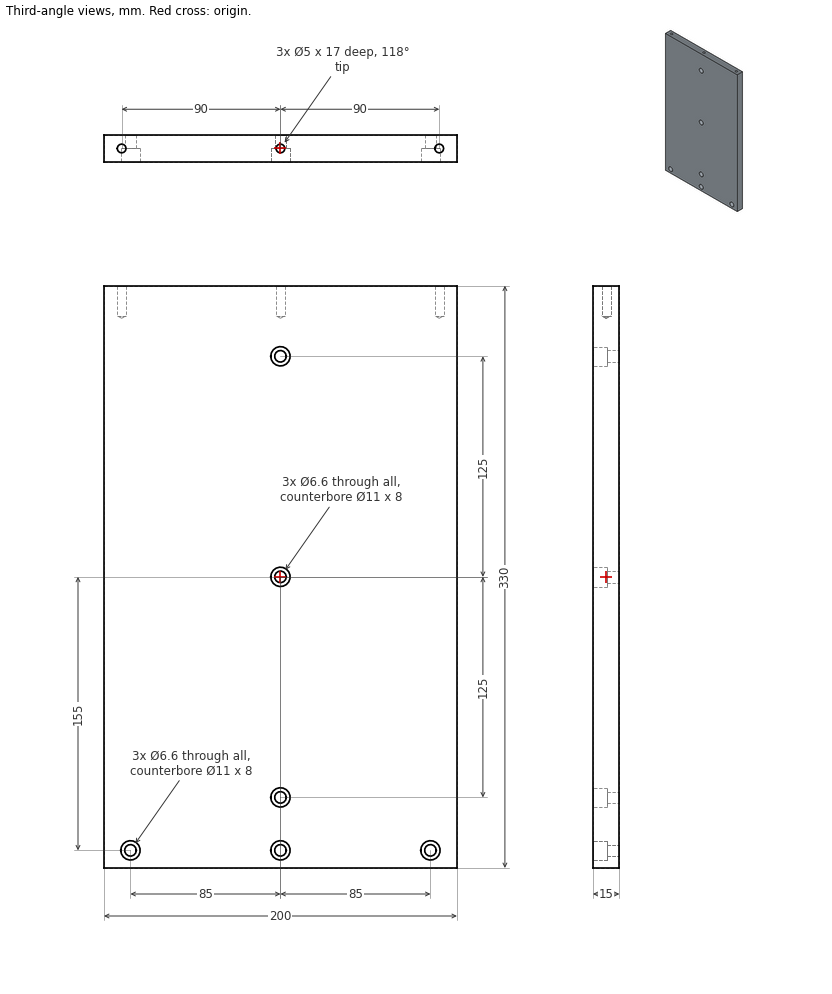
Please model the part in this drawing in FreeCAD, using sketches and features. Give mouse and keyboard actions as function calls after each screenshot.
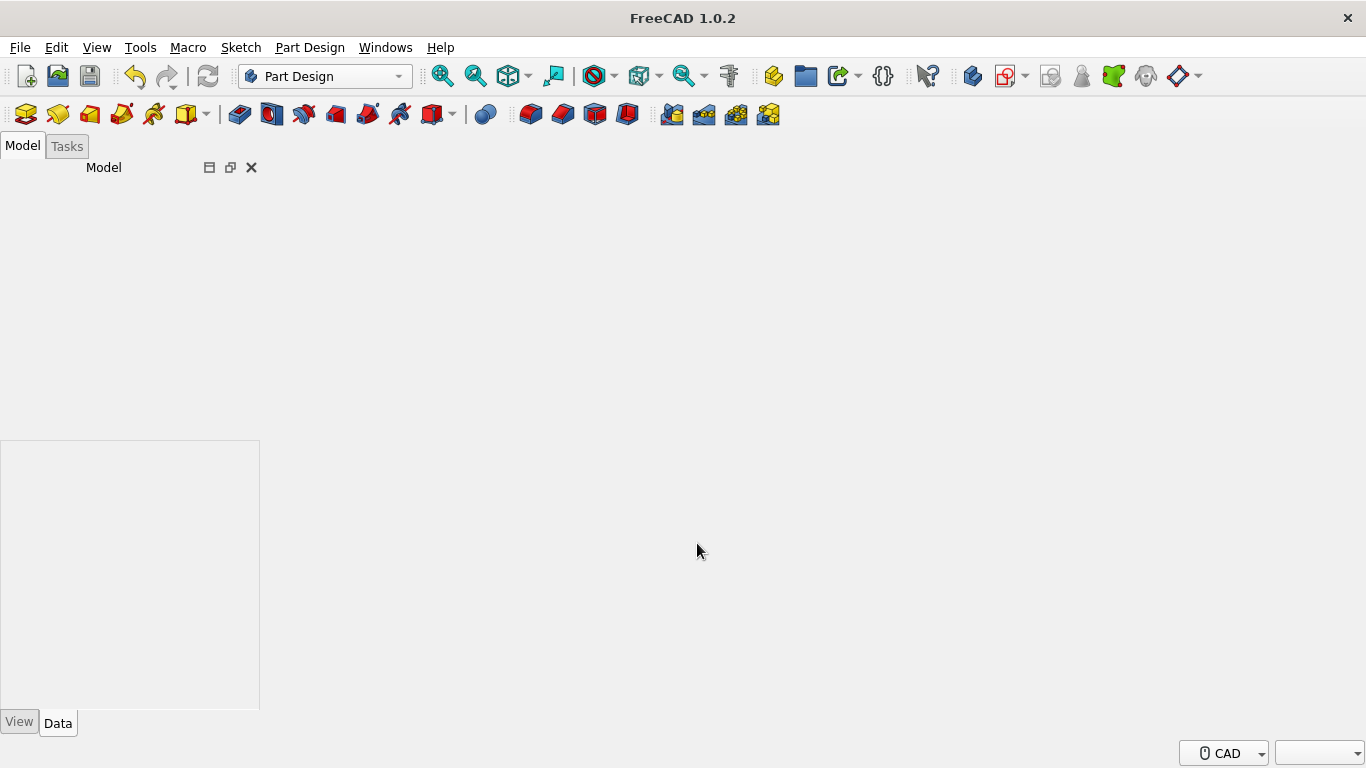
key(ctrl+n)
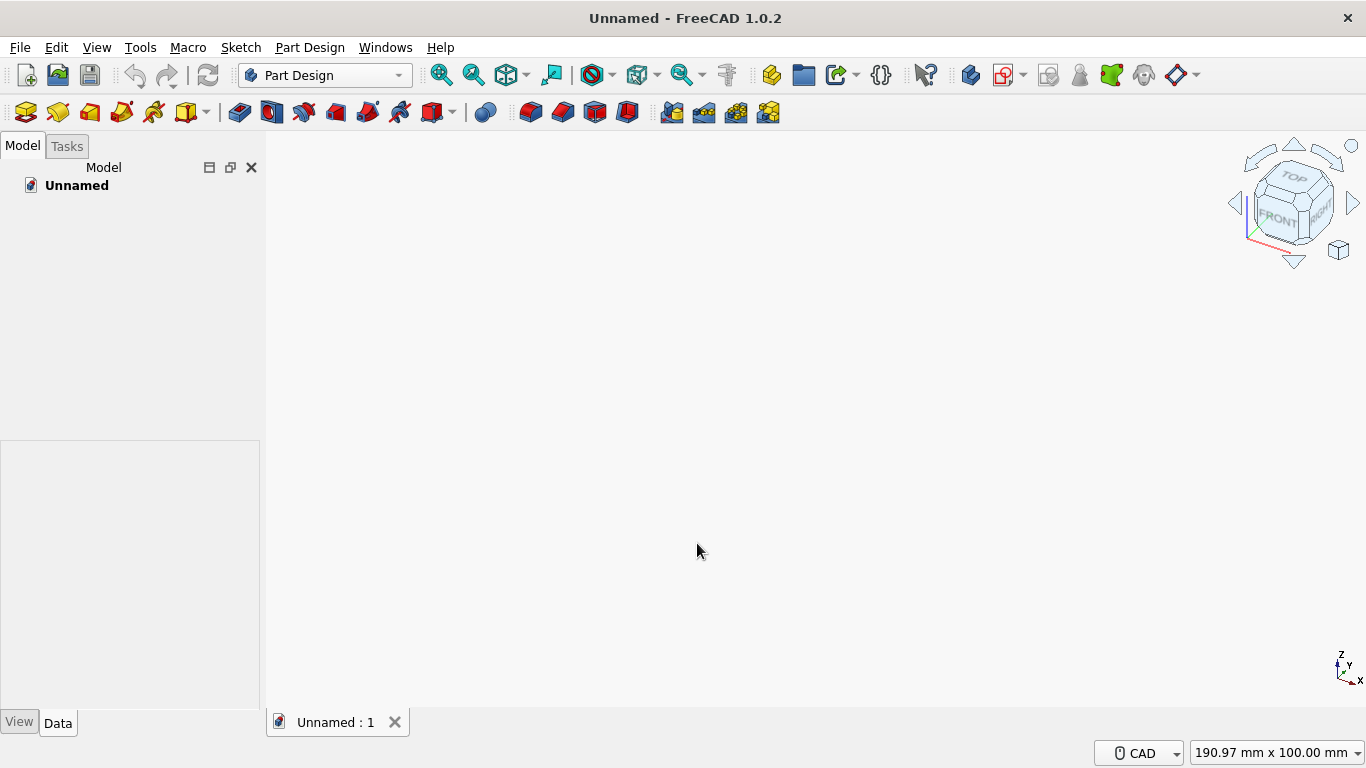
click(1004, 76)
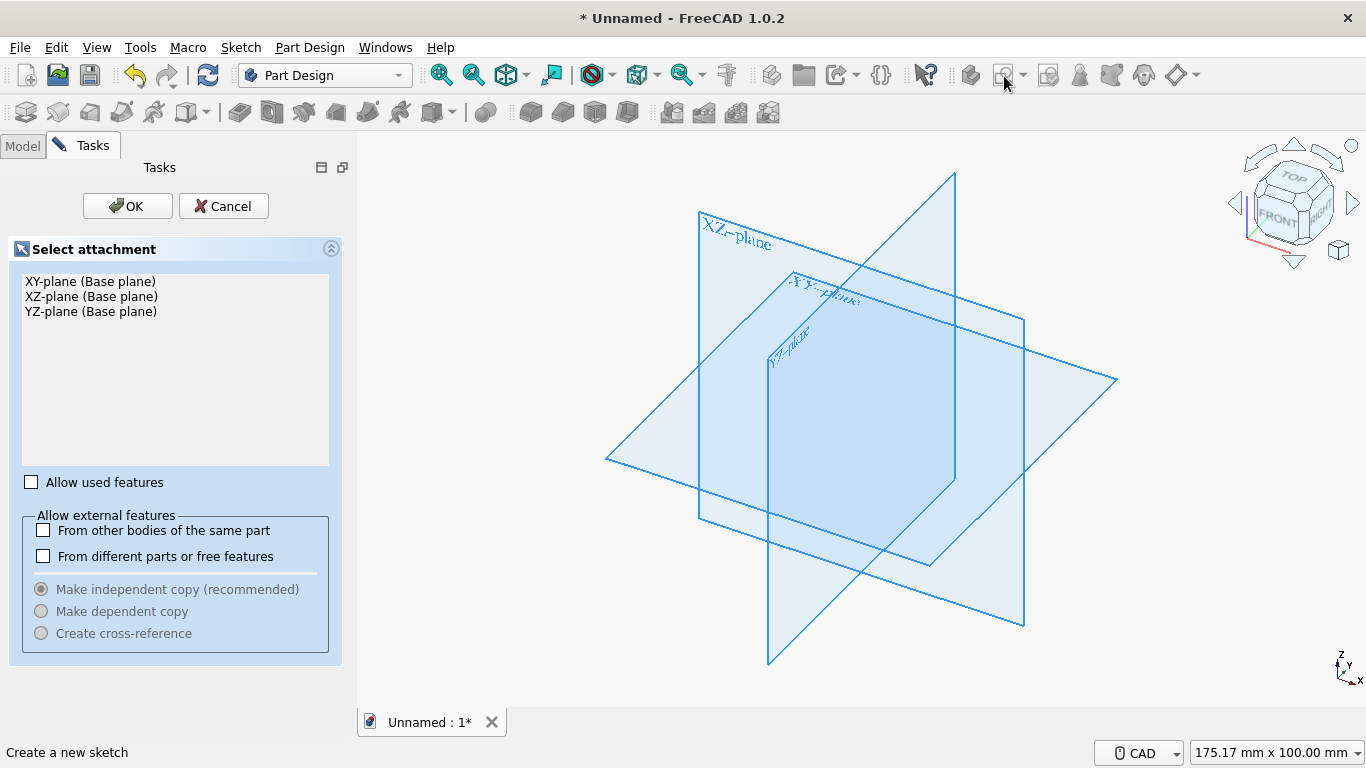
click(82, 296)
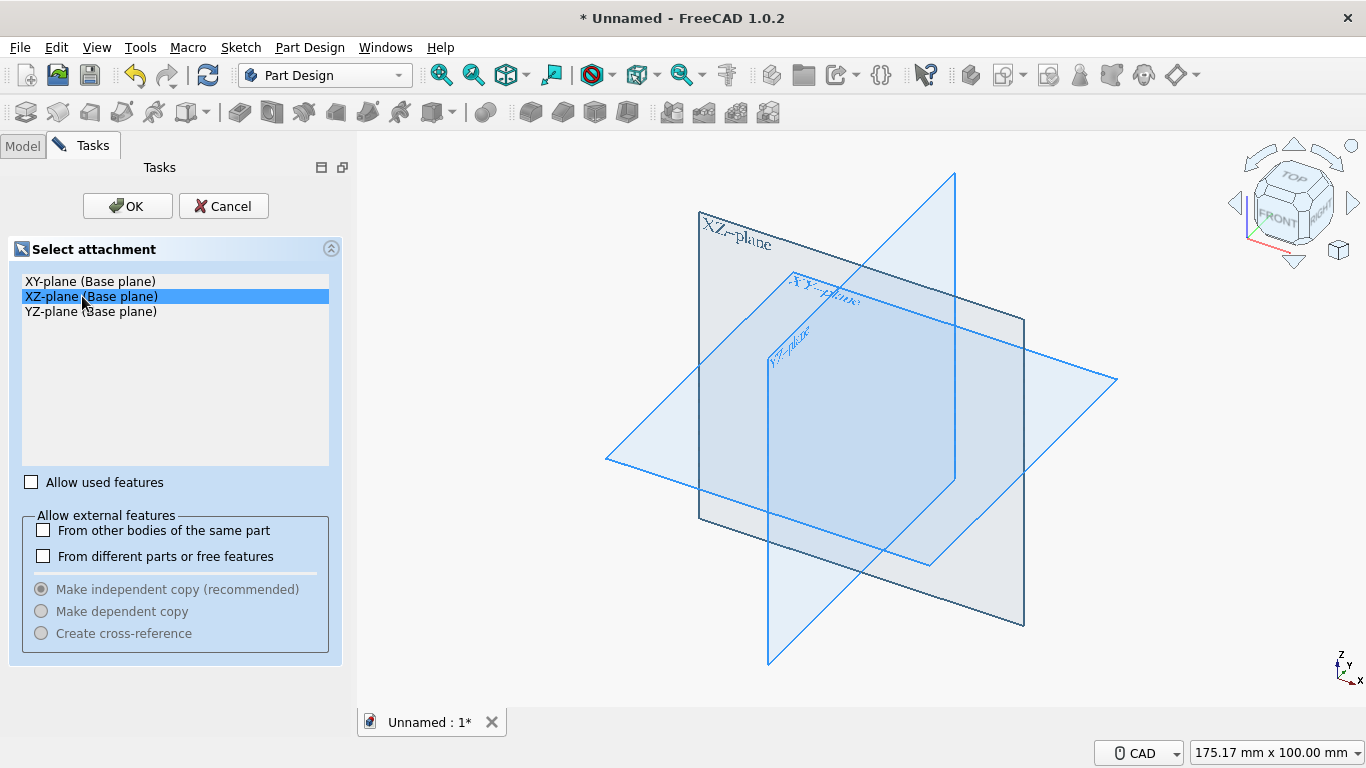
click(128, 206)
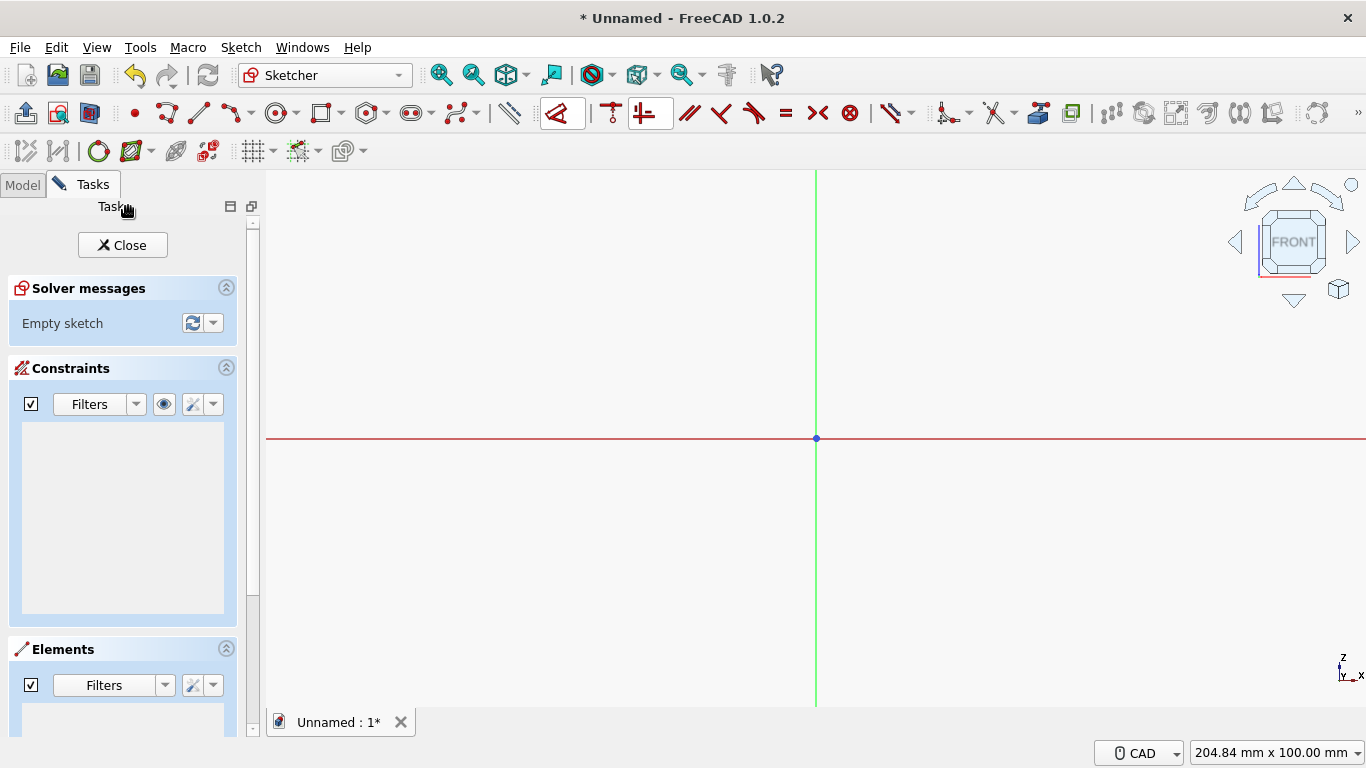
scroll(730, 438, down, 8)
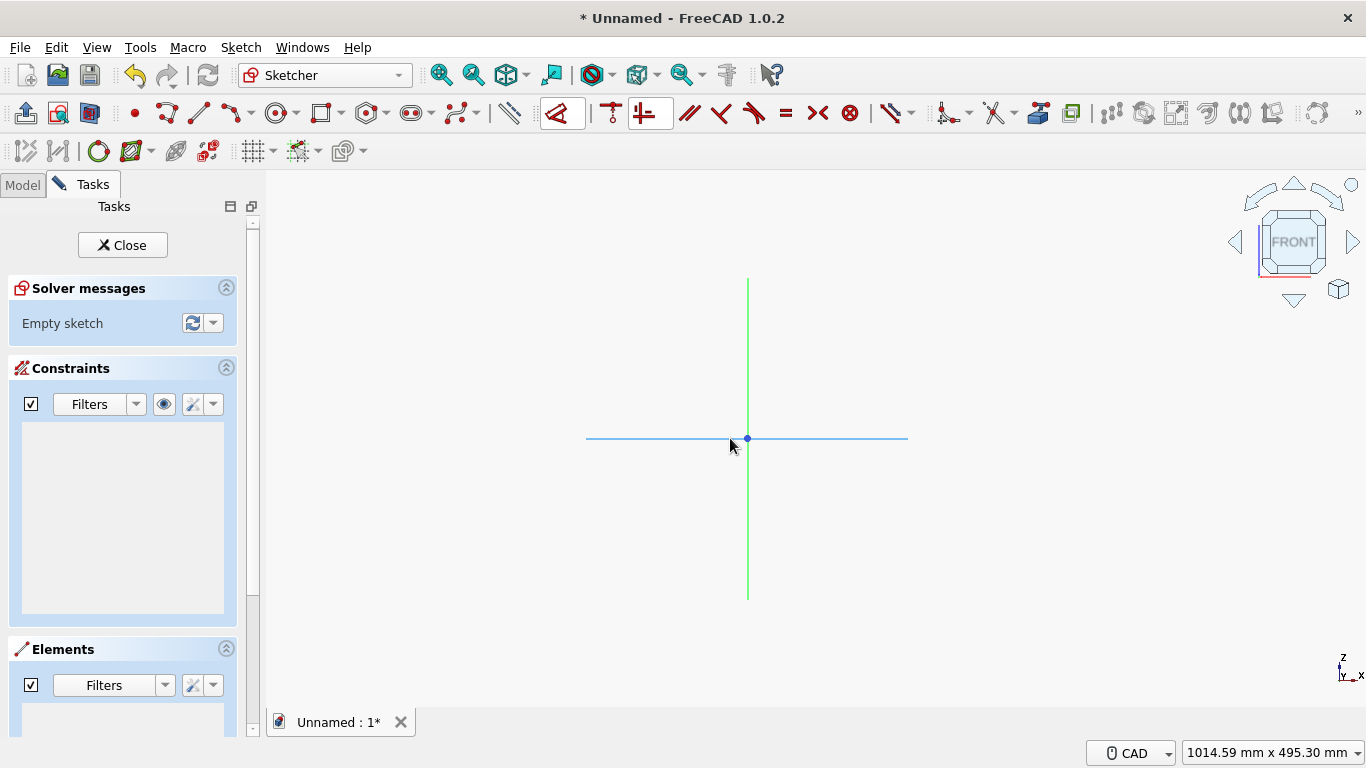
key(g)
key(v)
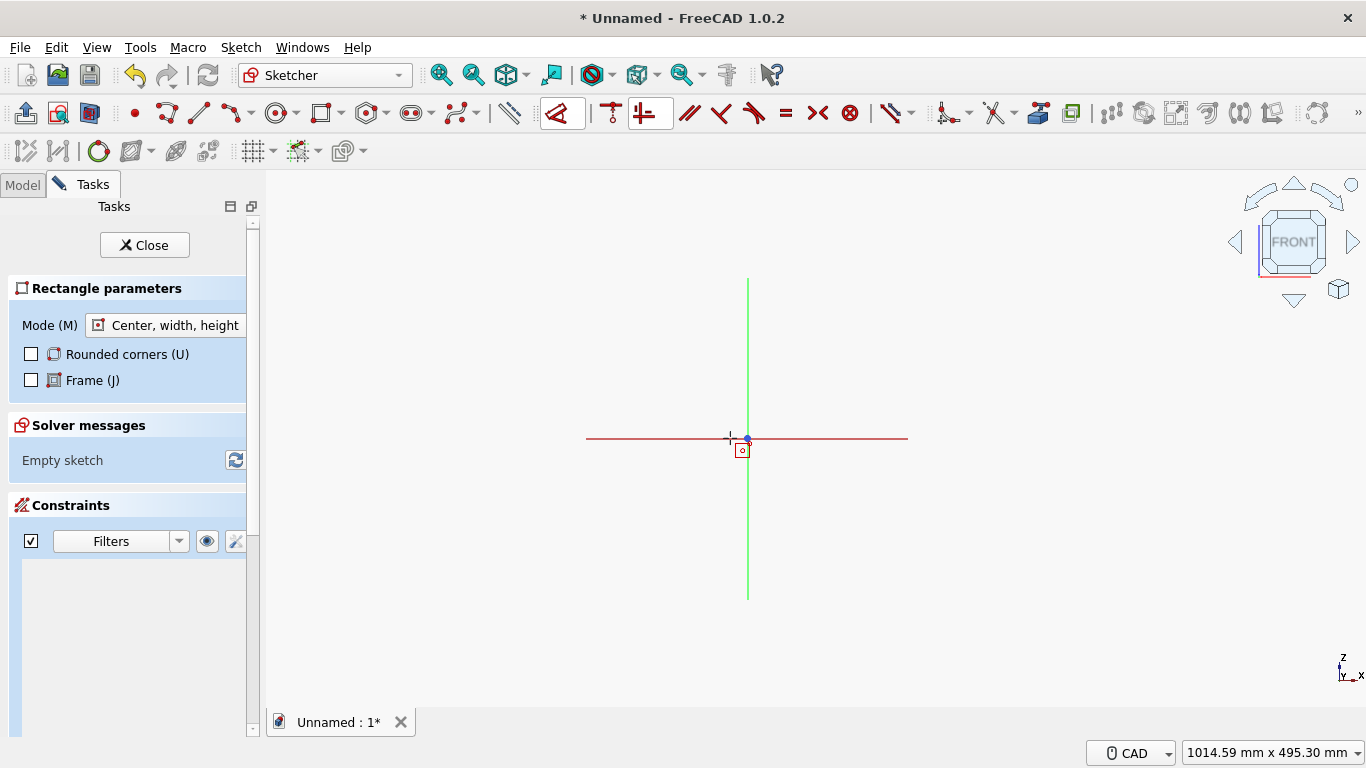
click(748, 438)
click(856, 260)
key(Escape)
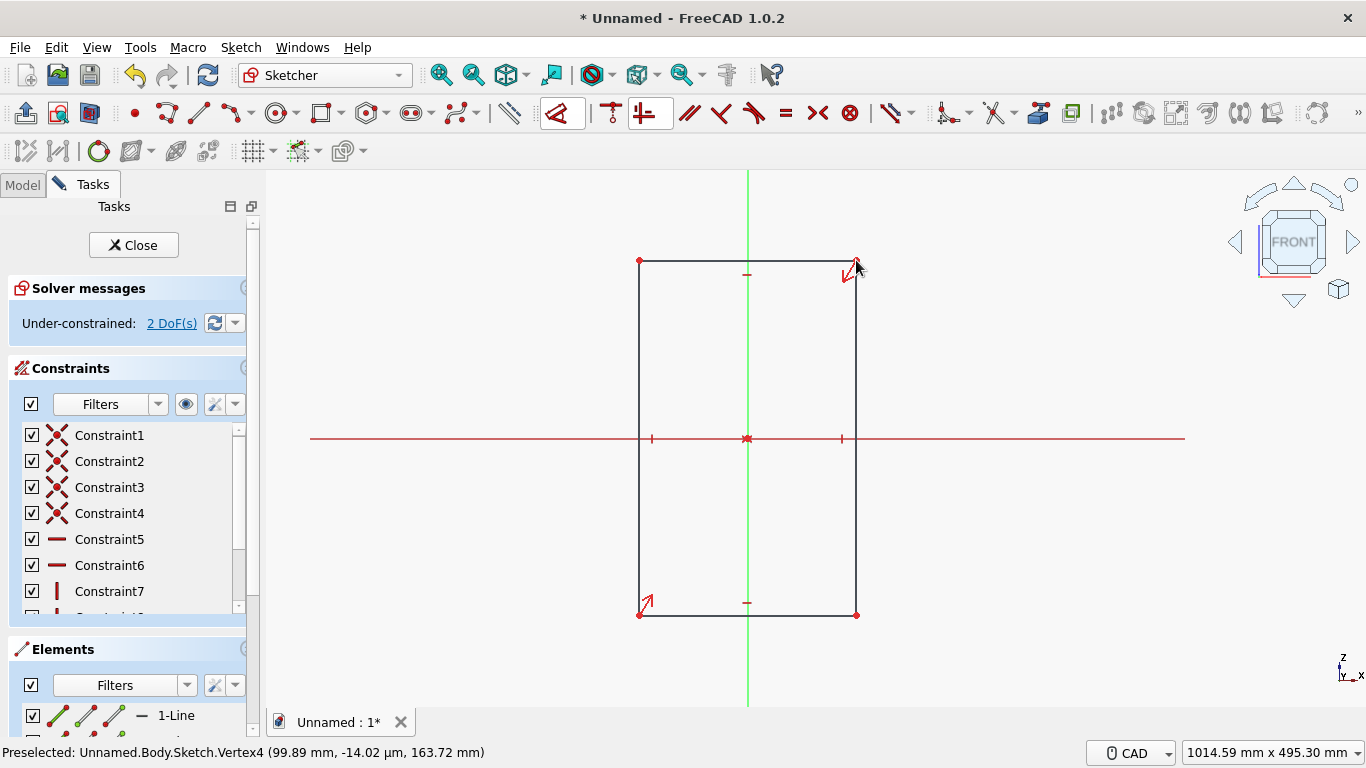
click(556, 114)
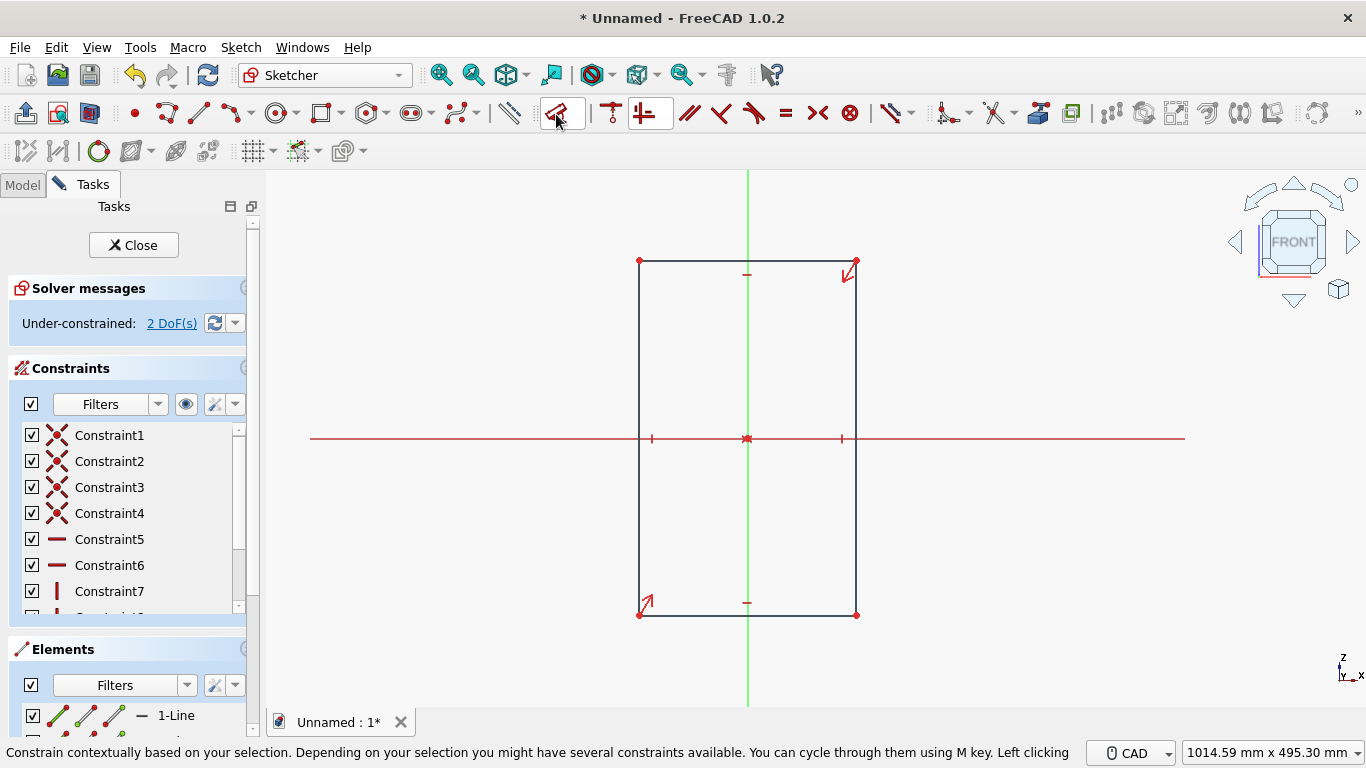
click(704, 616)
click(698, 650)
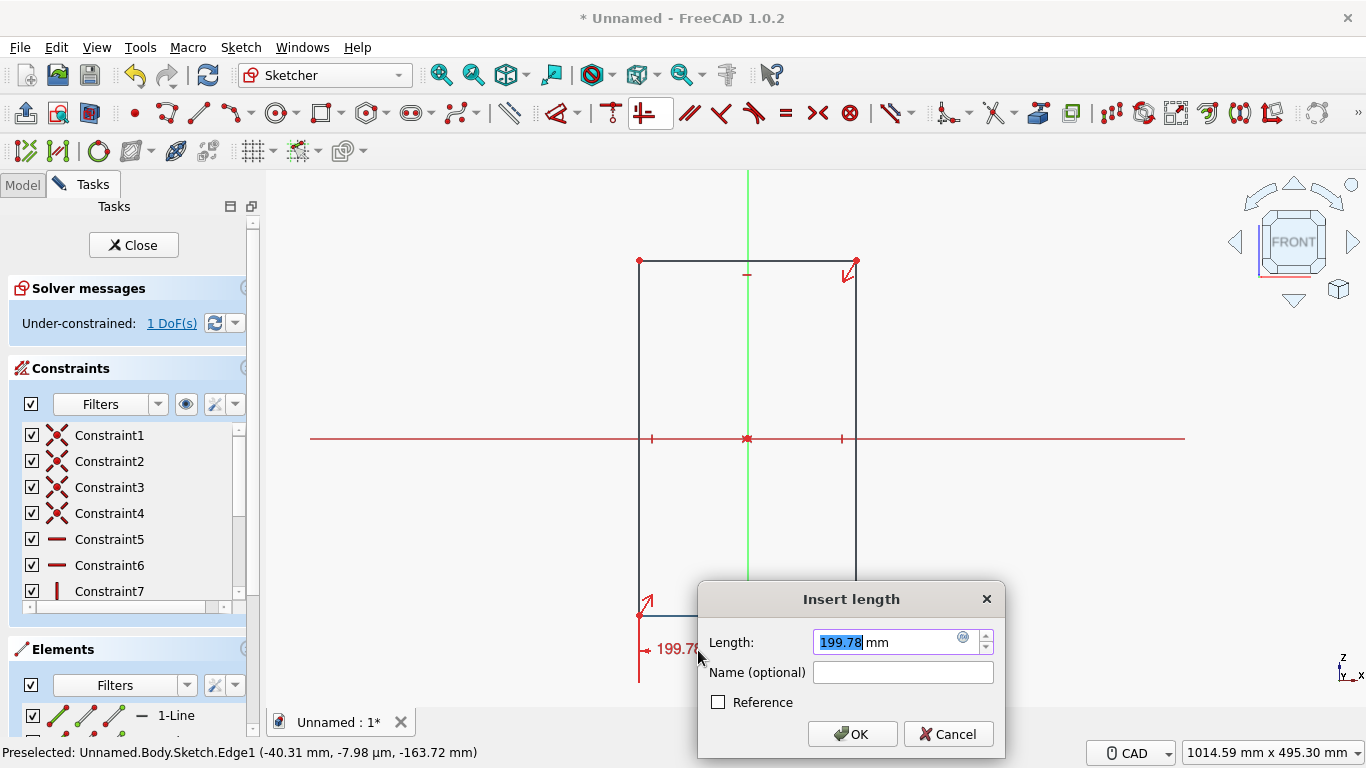
text(200)
key(Return)